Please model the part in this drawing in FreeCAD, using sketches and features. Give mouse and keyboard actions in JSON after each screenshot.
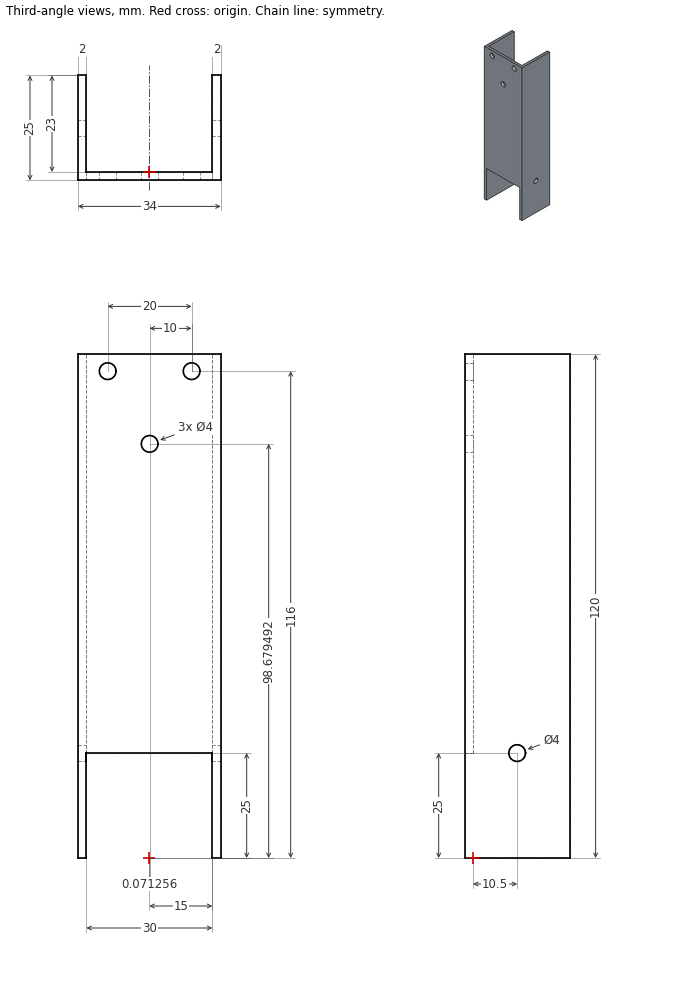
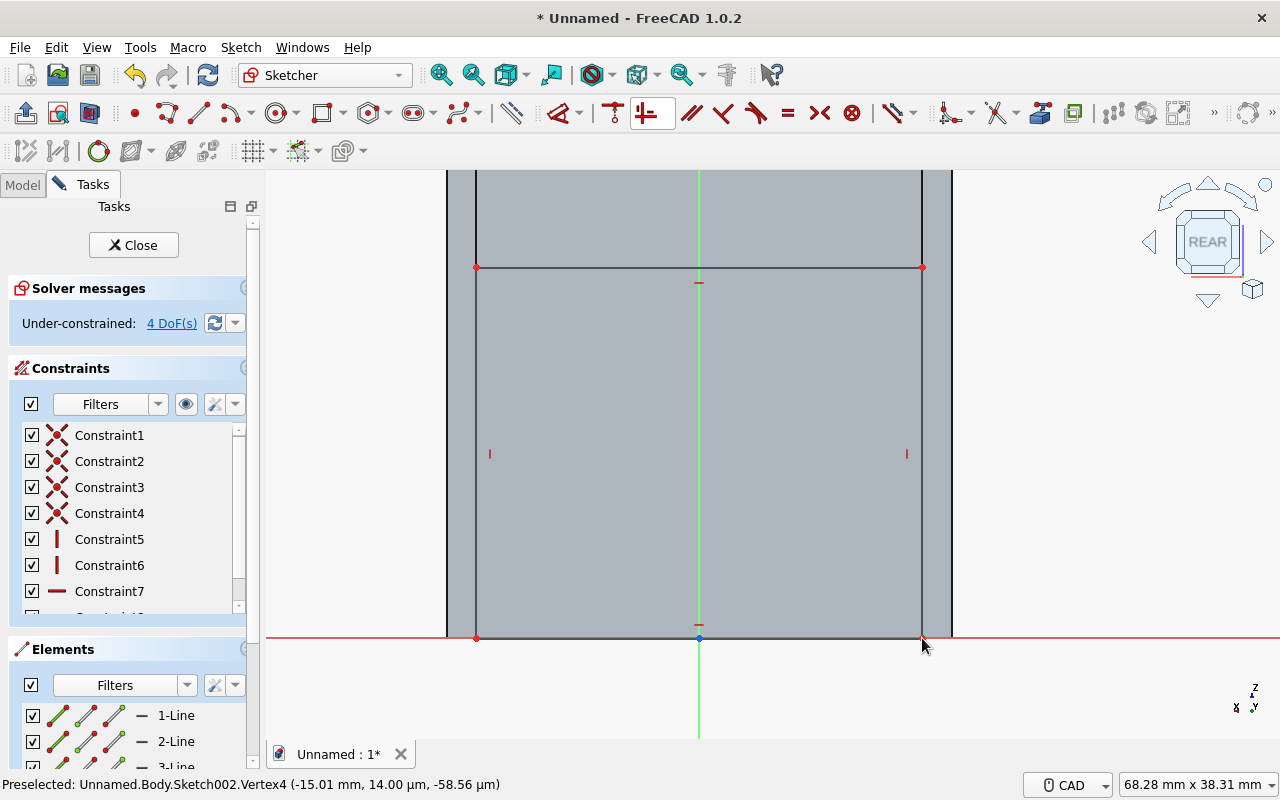
{"action": "left_click", "coordinate": [476, 639]}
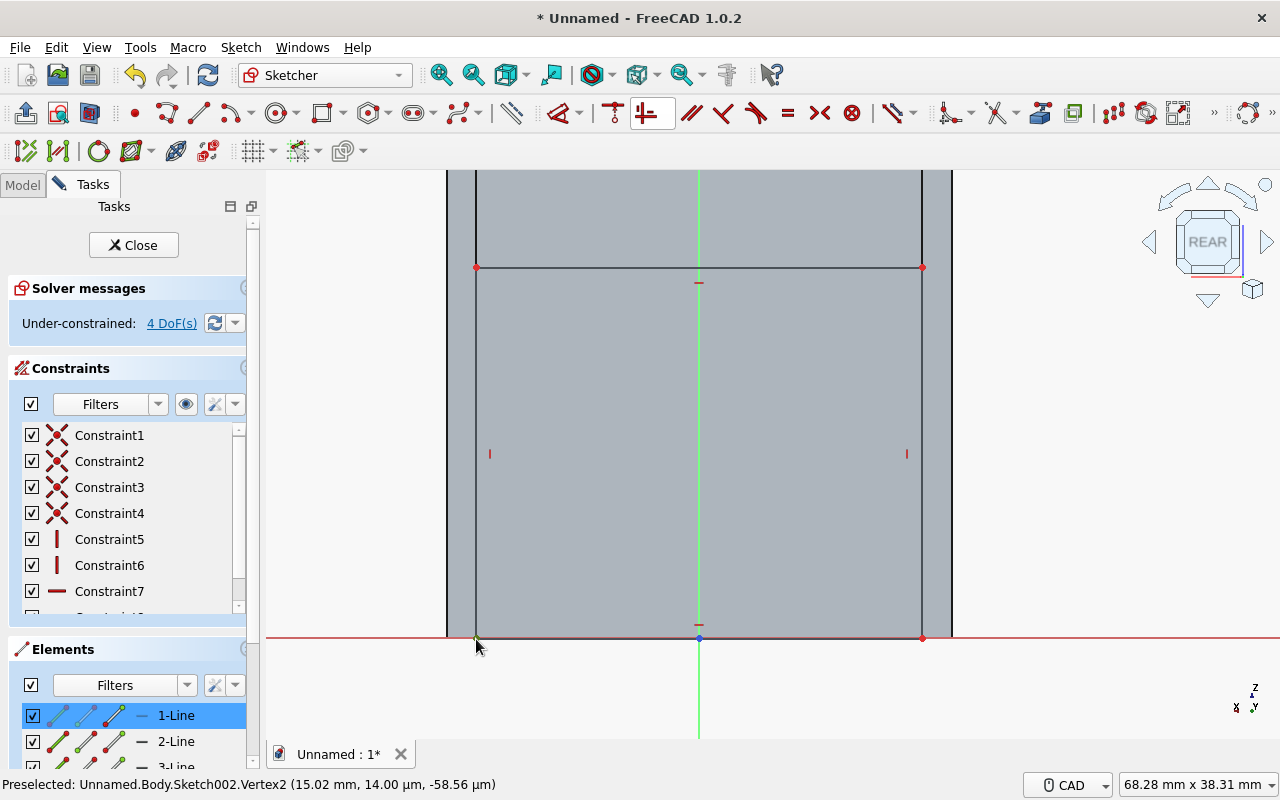
{"action": "left_click", "coordinate": [353, 638]}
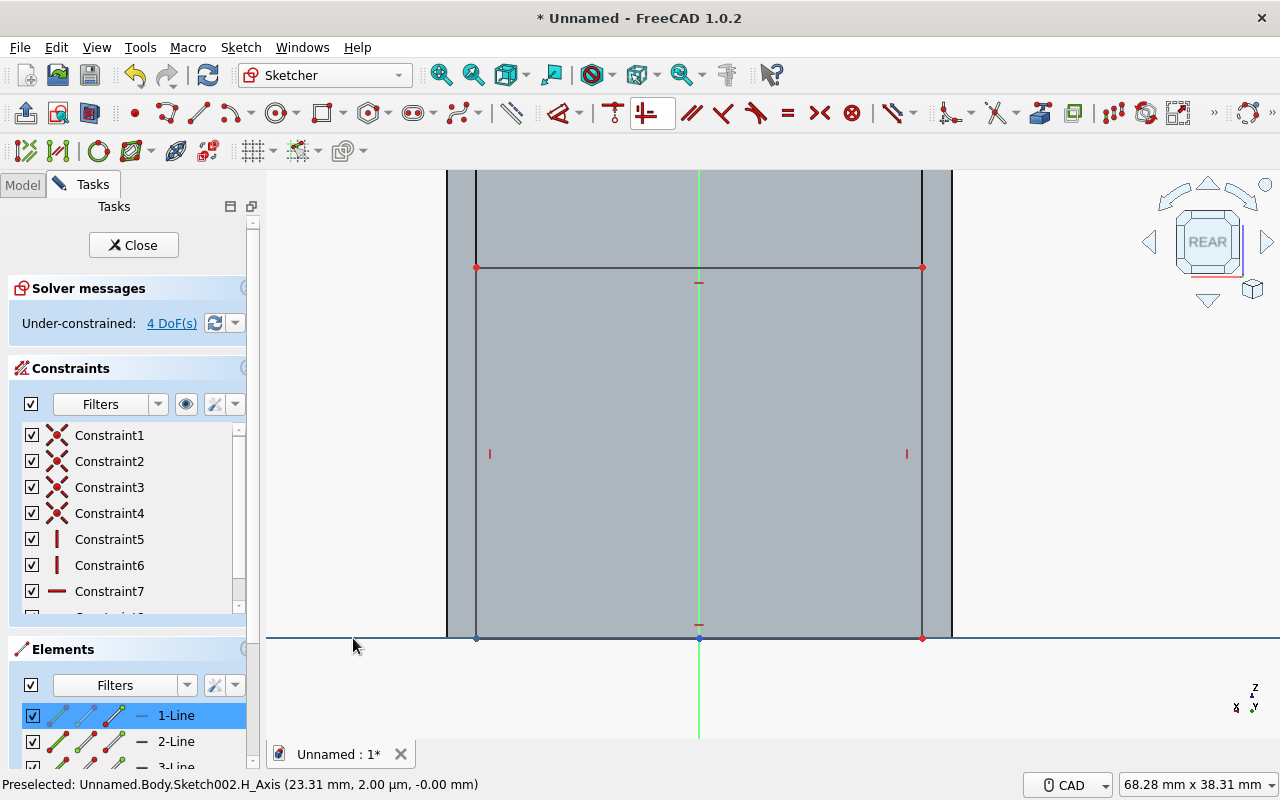
{"action": "left_click", "coordinate": [614, 114]}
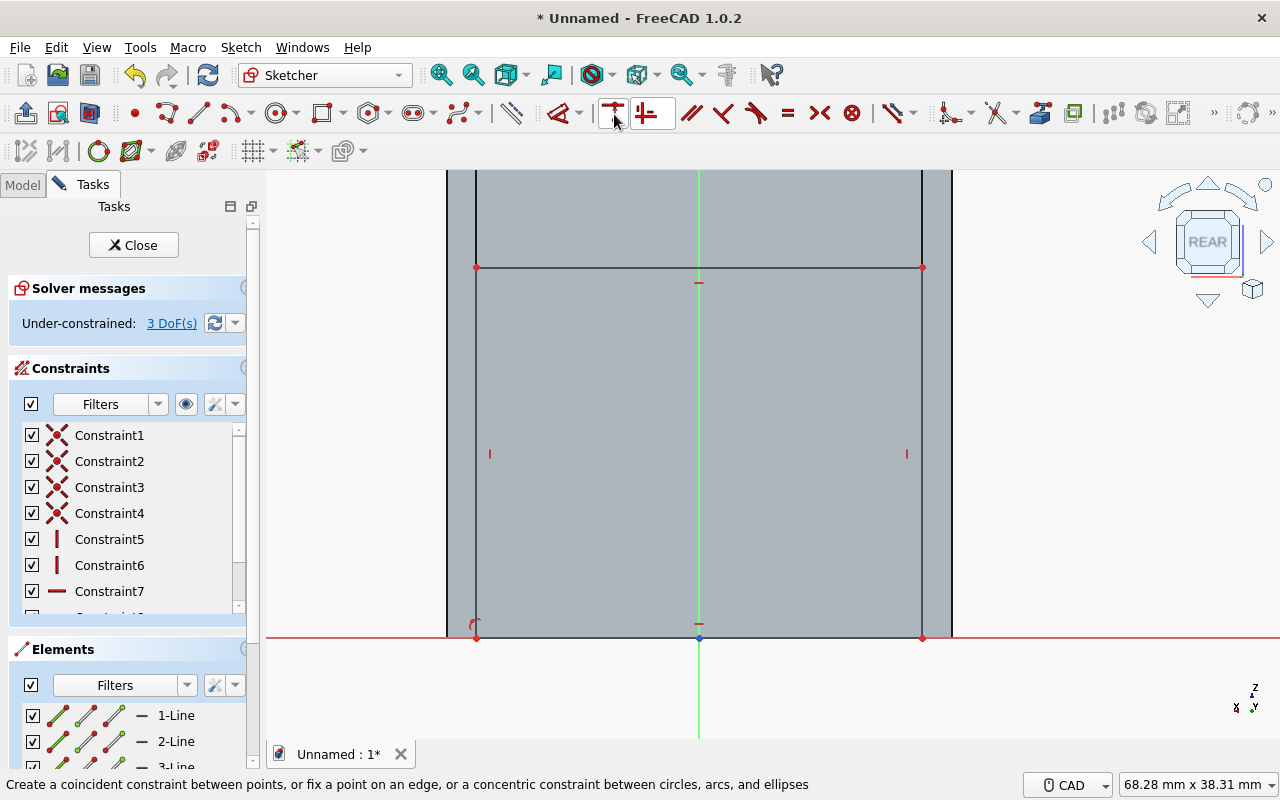
{"action": "left_click", "coordinate": [558, 114]}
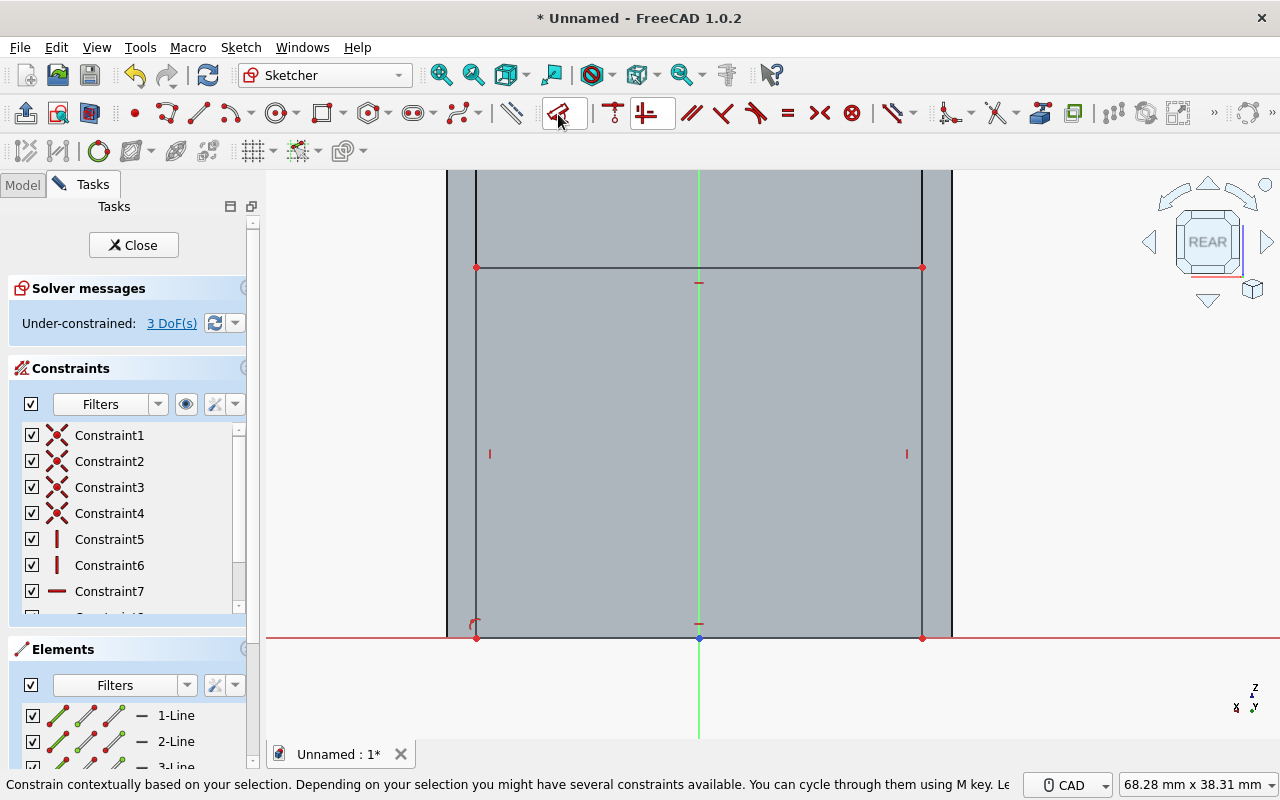
{"action": "left_click", "coordinate": [476, 379]}
{"action": "left_click", "coordinate": [442, 453]}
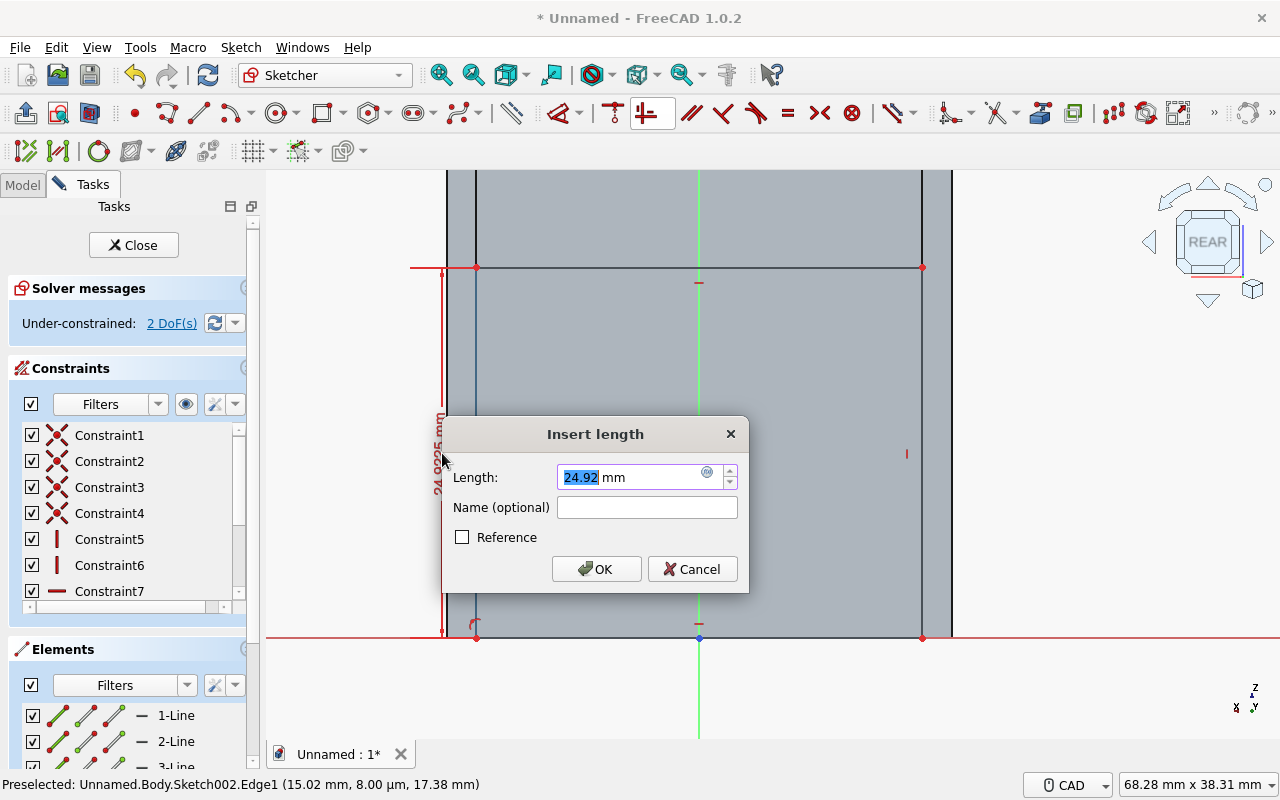
{"action": "type", "text": "25"}
{"action": "key", "text": "Return"}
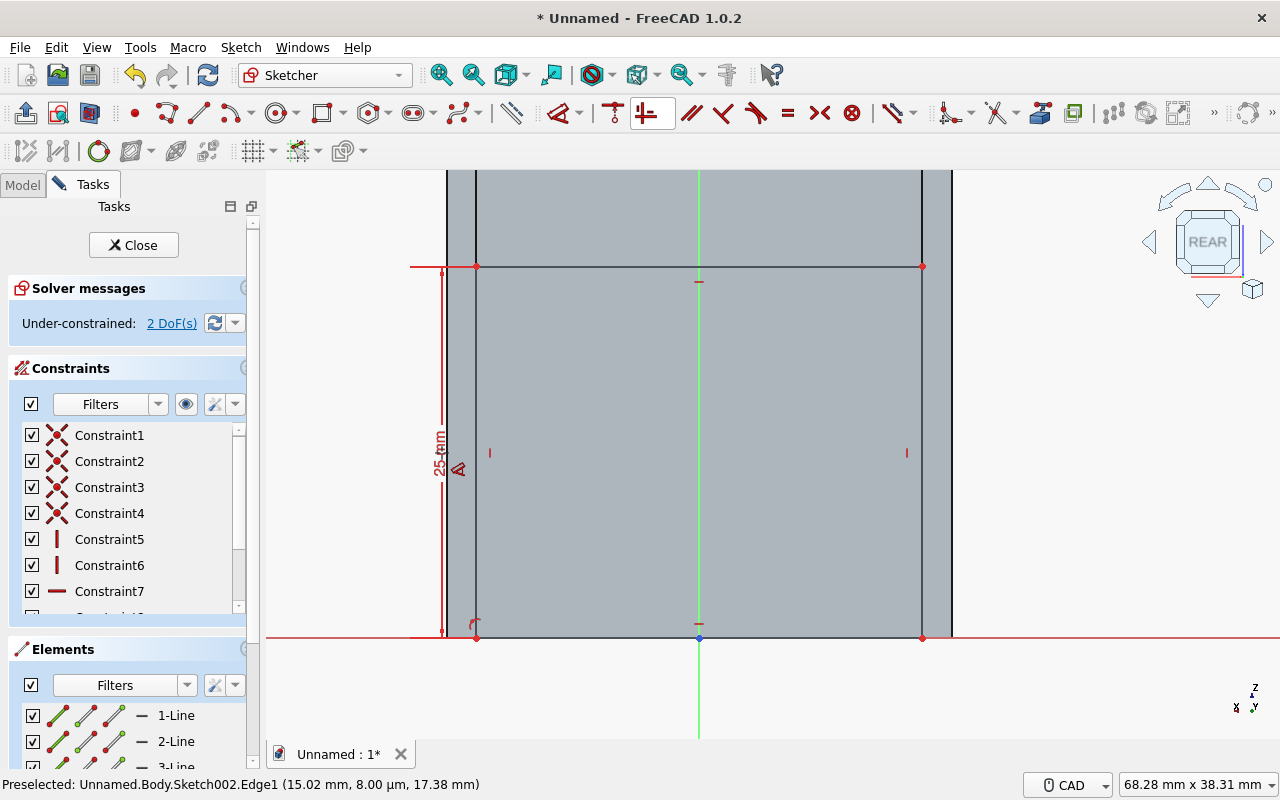
{"action": "left_click", "coordinate": [610, 638]}
{"action": "left_click", "coordinate": [596, 672]}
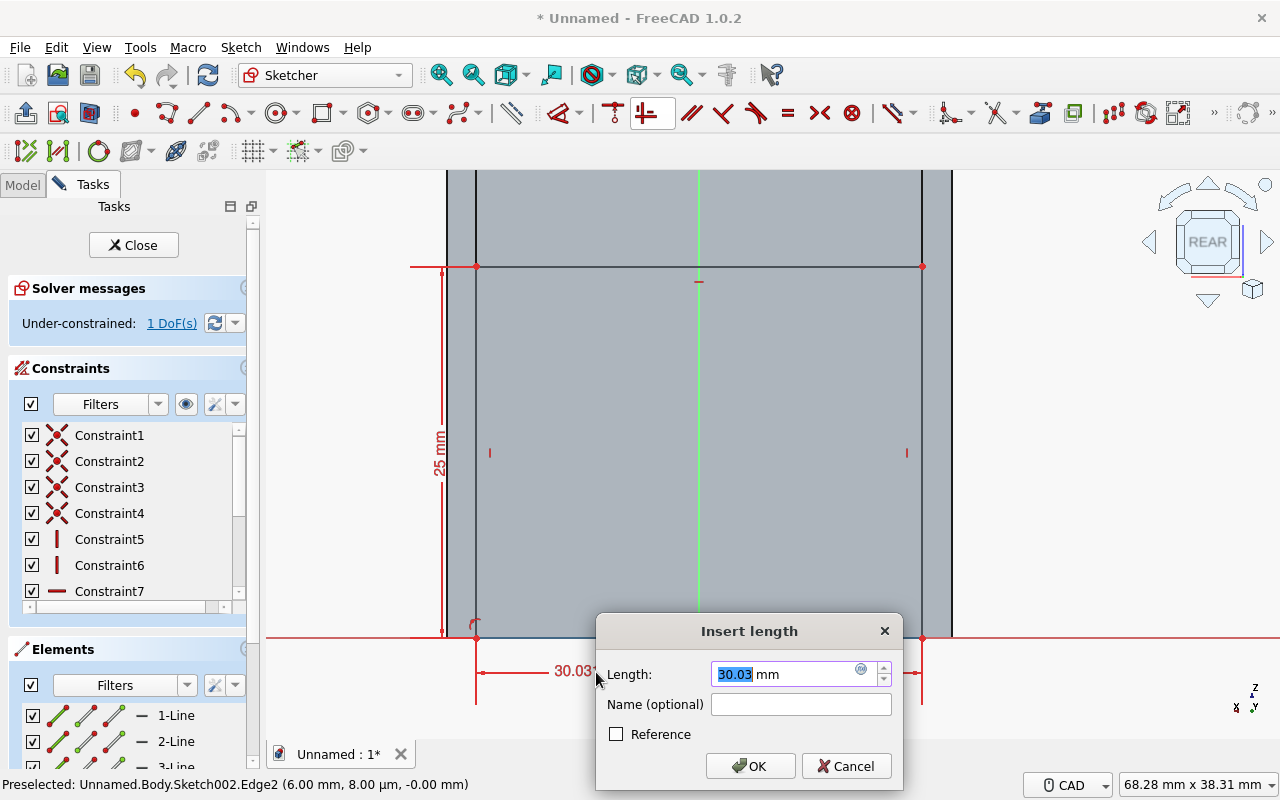
{"action": "type", "text": "30"}
{"action": "key", "text": "Return"}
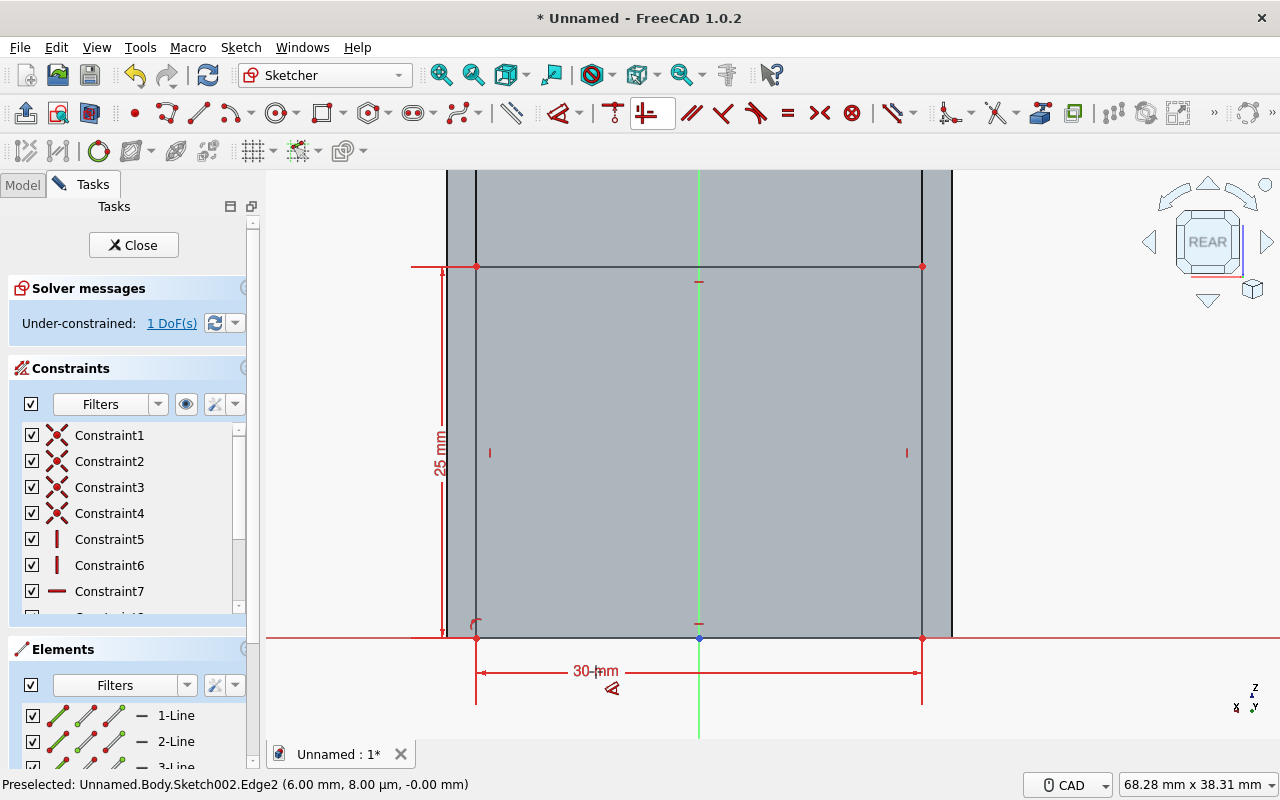
{"action": "left_click", "coordinate": [476, 267]}
{"action": "left_click", "coordinate": [510, 672]}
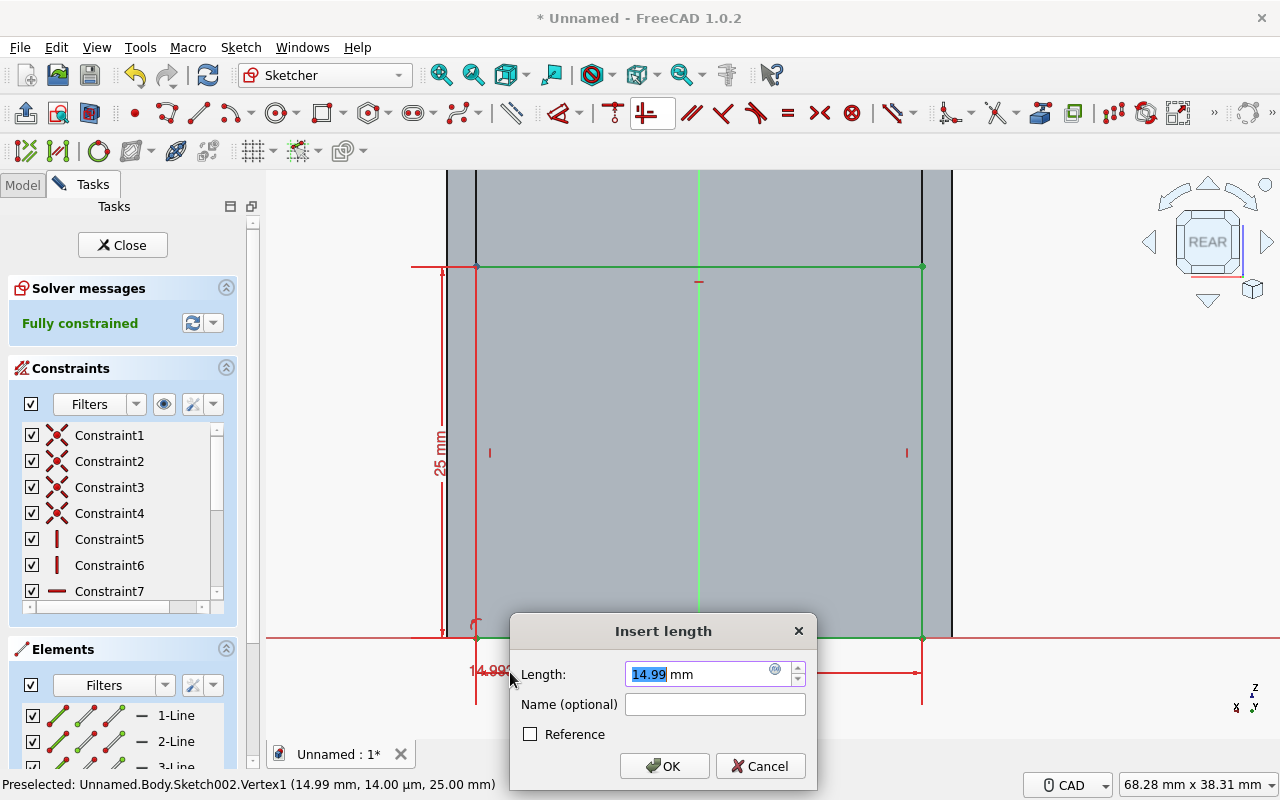
{"action": "type", "text": "15"}
{"action": "key", "text": "Return"}
{"action": "key", "text": "Escape"}